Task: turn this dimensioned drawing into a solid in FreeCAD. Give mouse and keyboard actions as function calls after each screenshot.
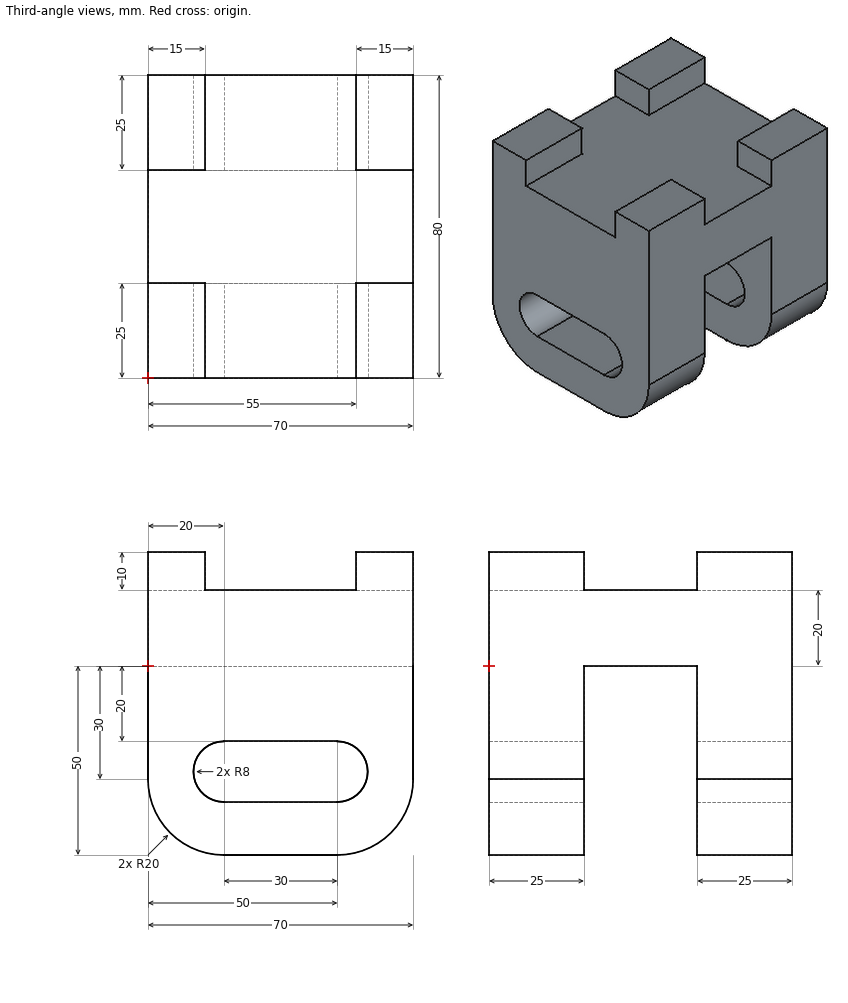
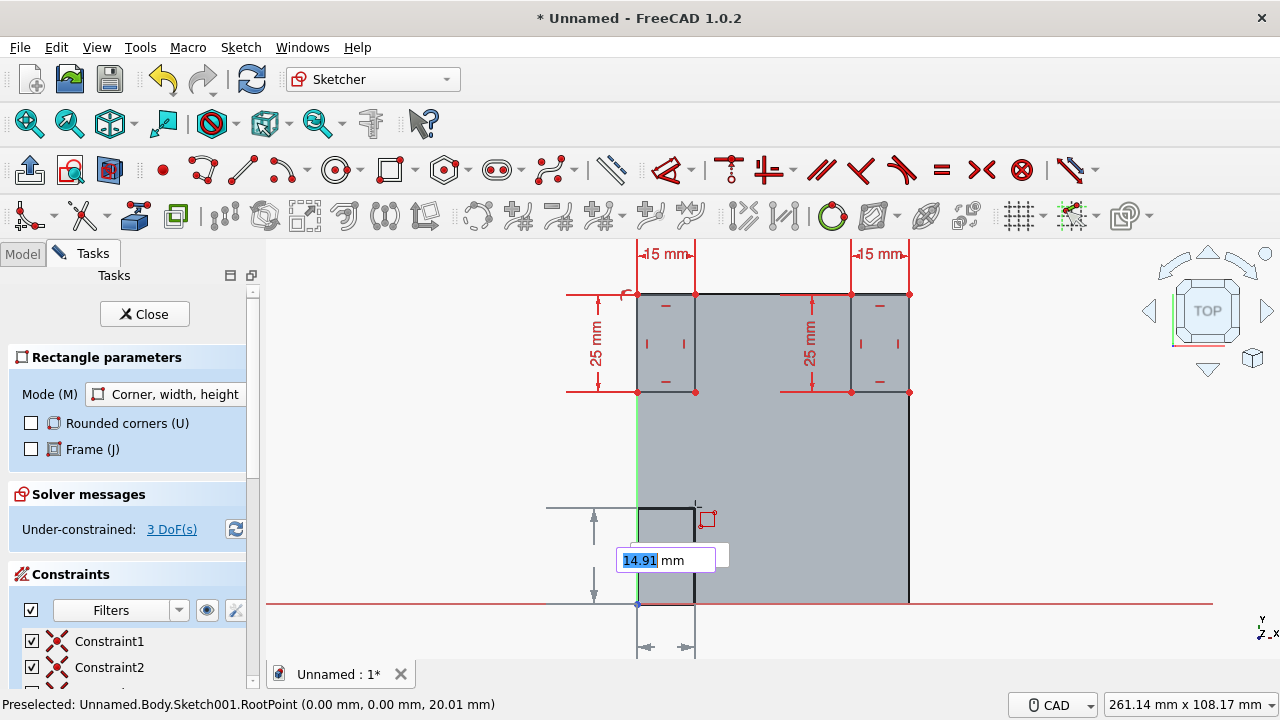
text(15)
key(Tab)
text(25)
key(Return)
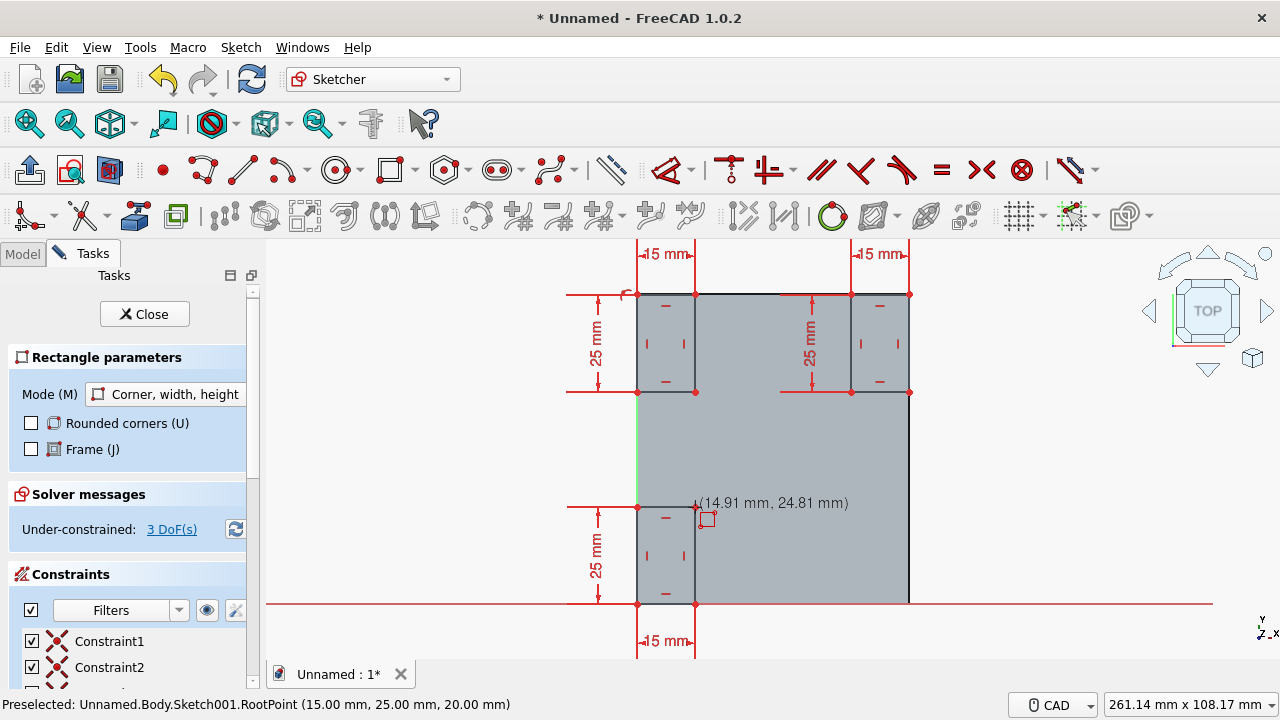
click(851, 507)
click(909, 604)
key(Escape)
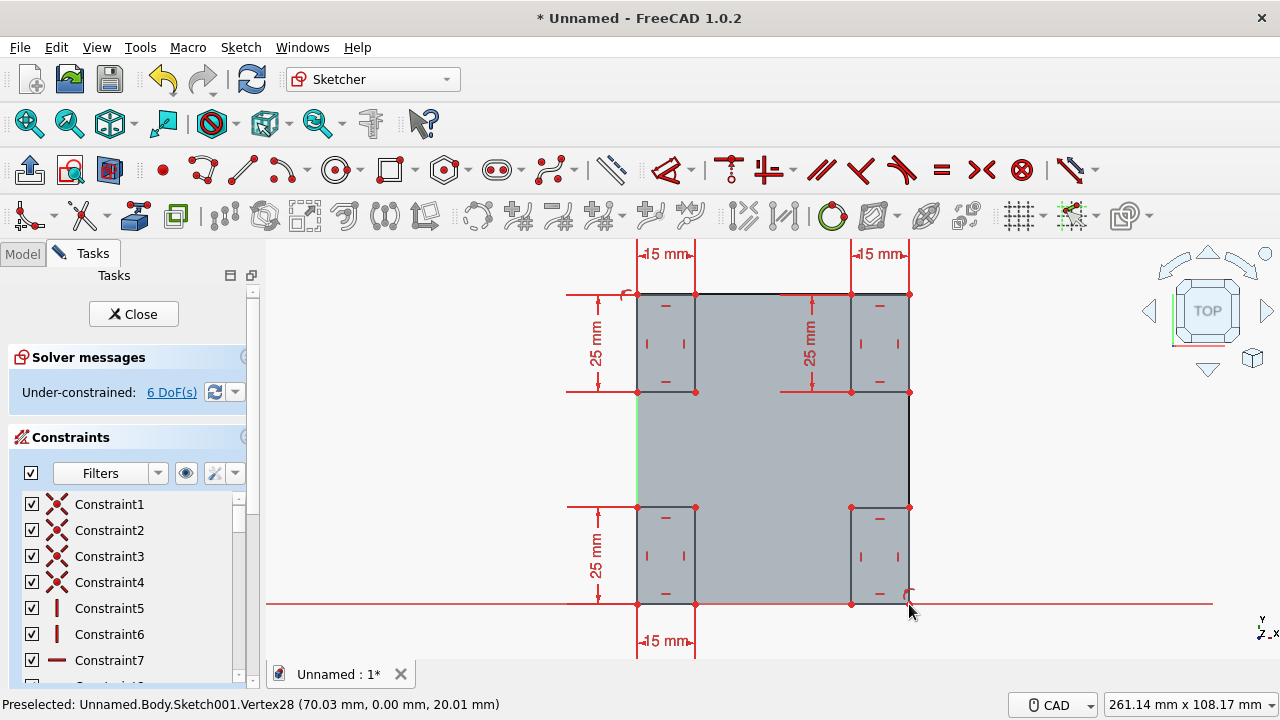
click(666, 170)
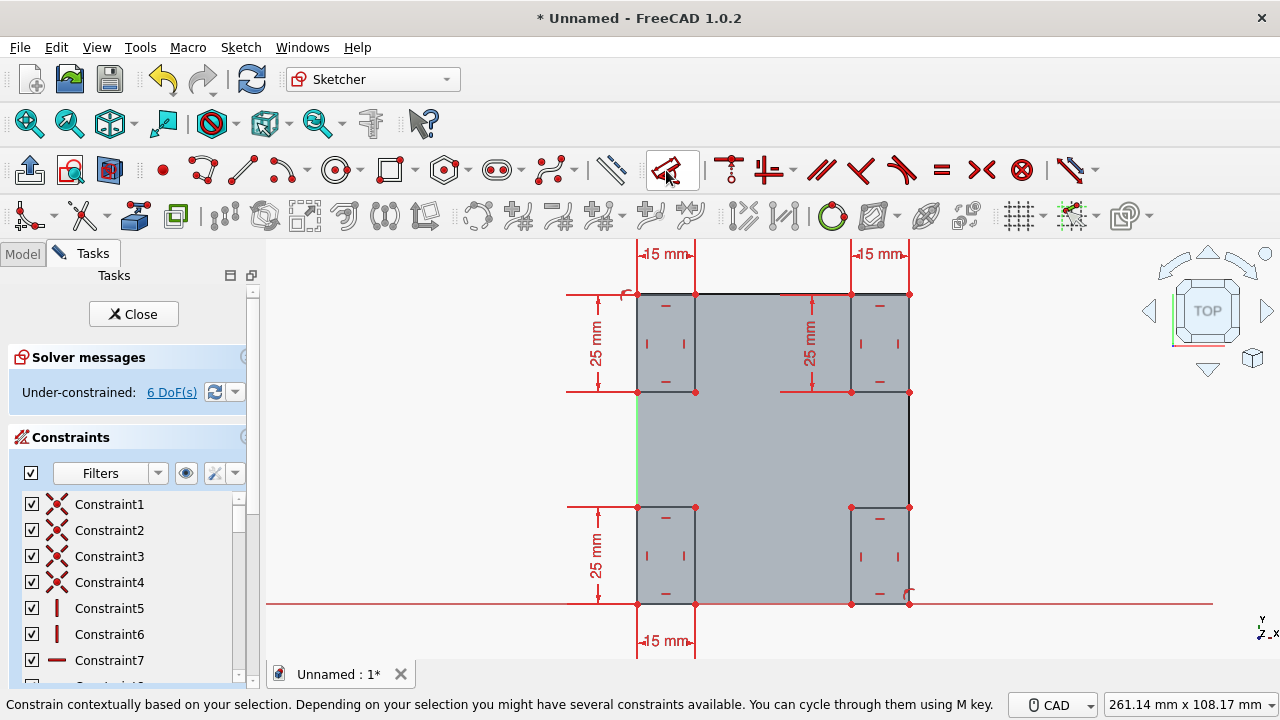
click(851, 537)
click(885, 556)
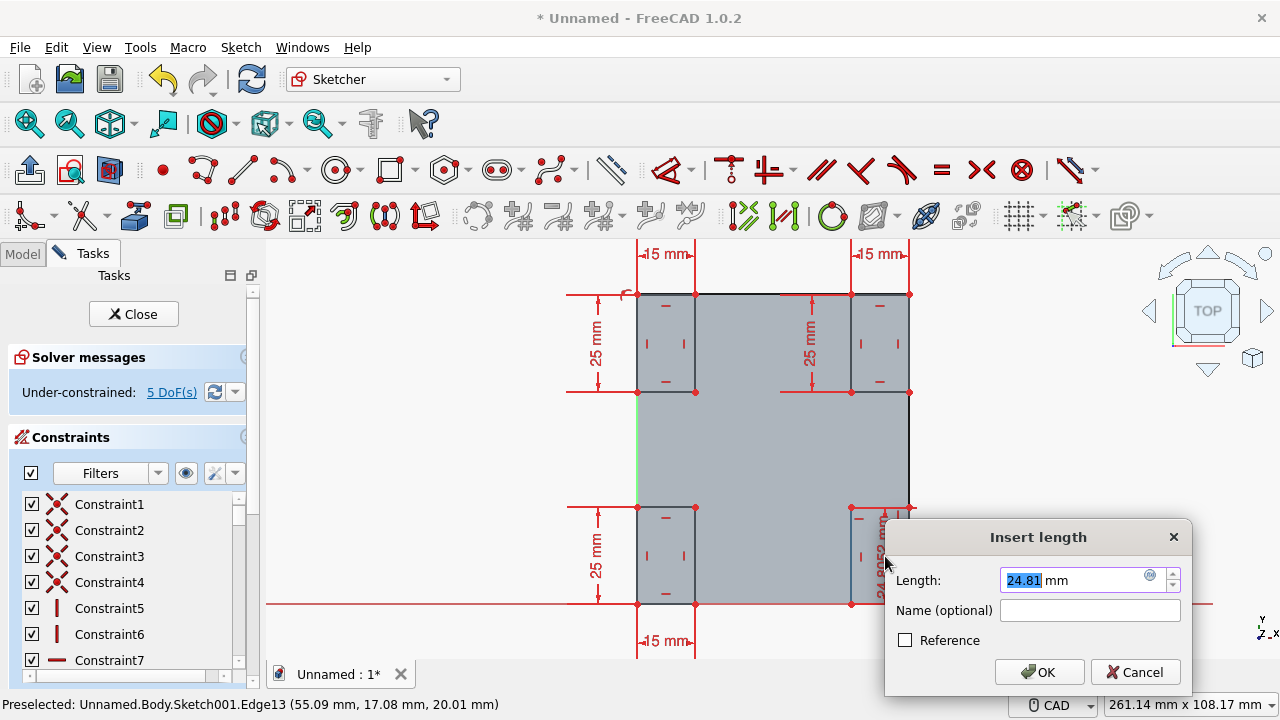
text(25)
key(Return)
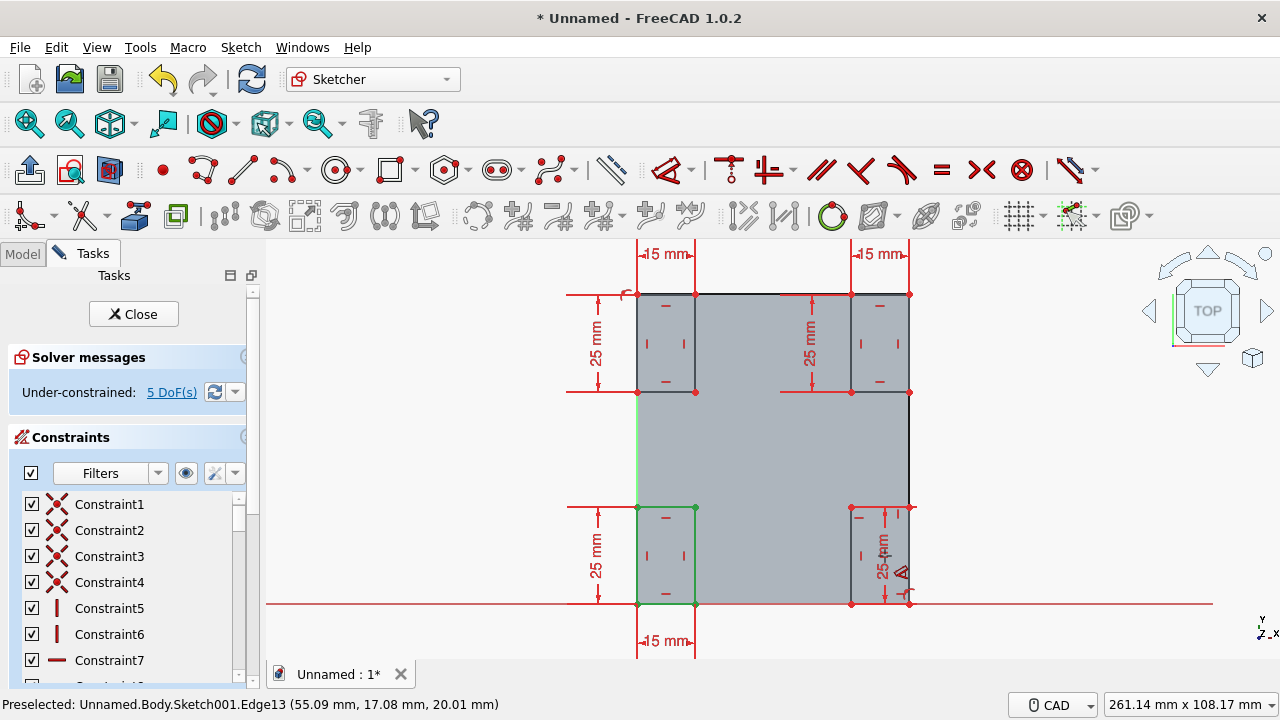
click(868, 604)
click(880, 522)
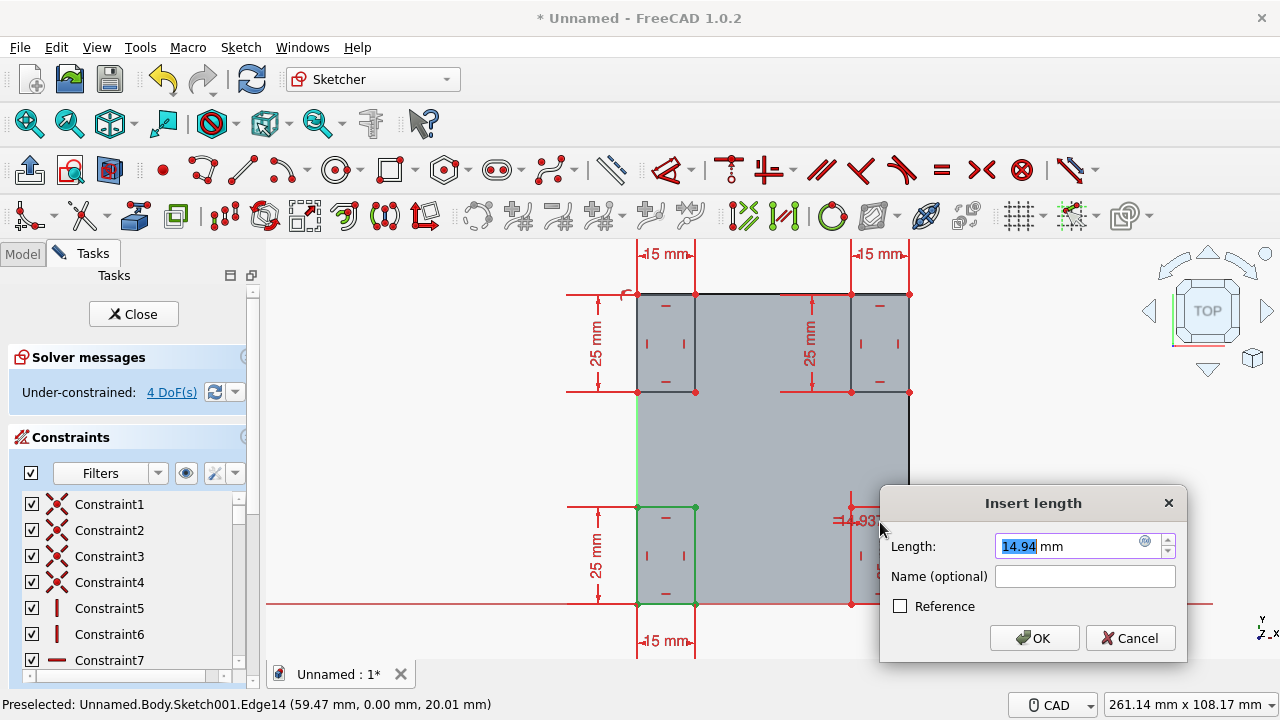
text(15)
key(Return)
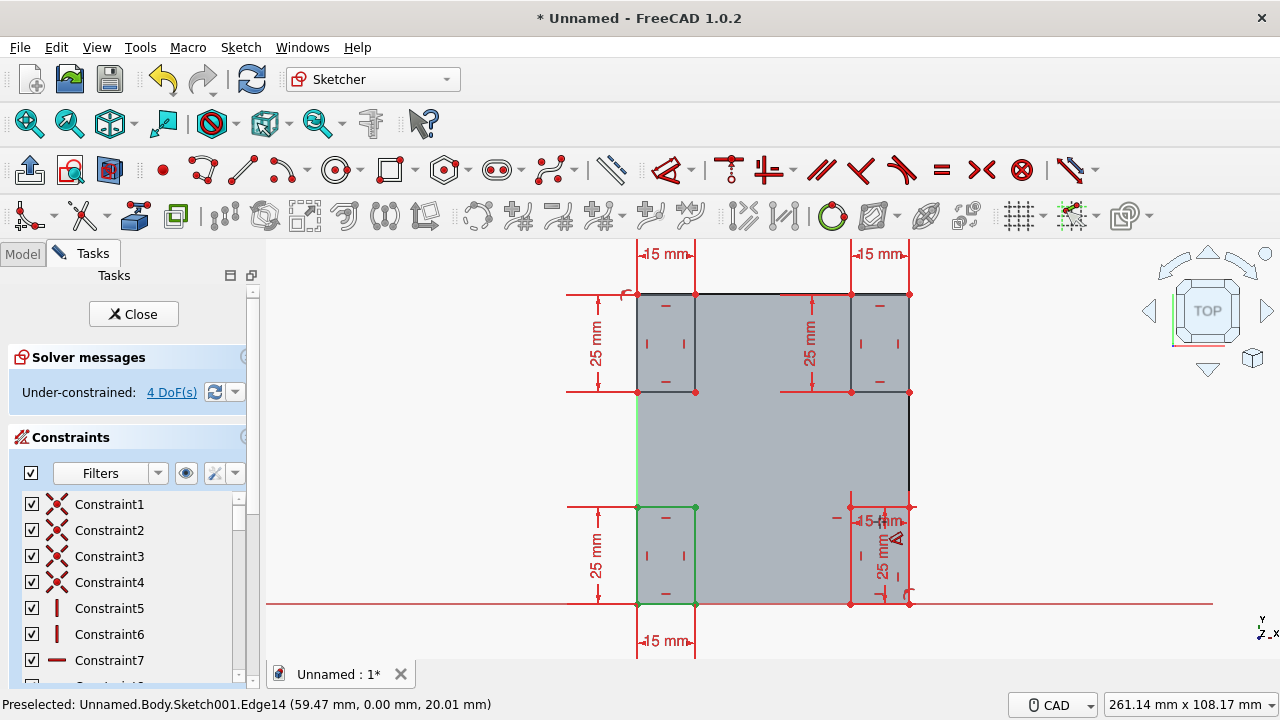
click(637, 295)
click(603, 450)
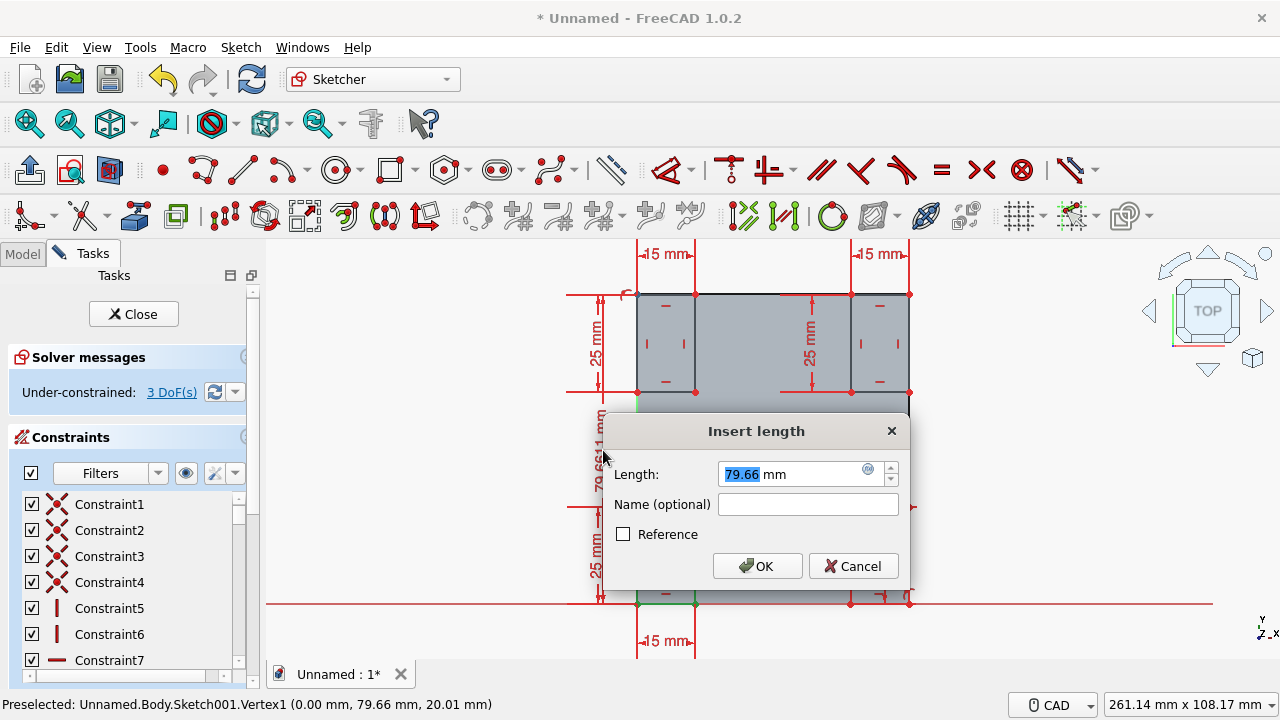
text(80)
key(Return)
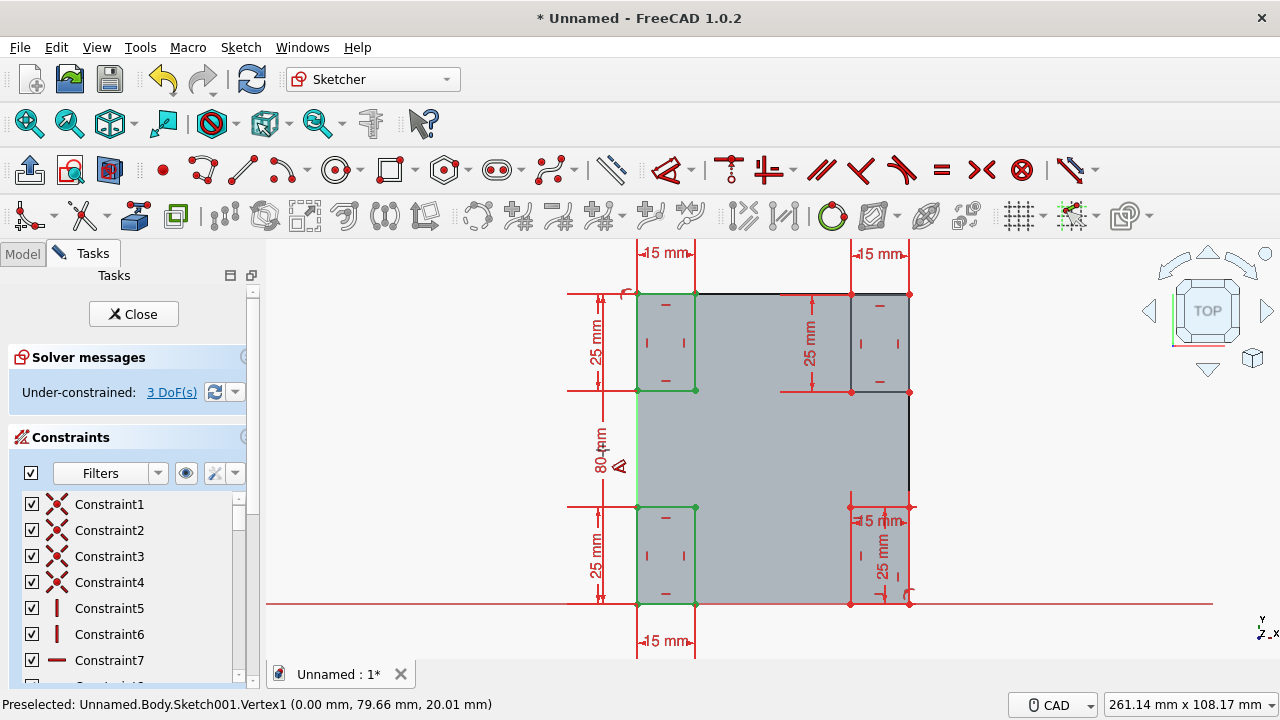
click(851, 295)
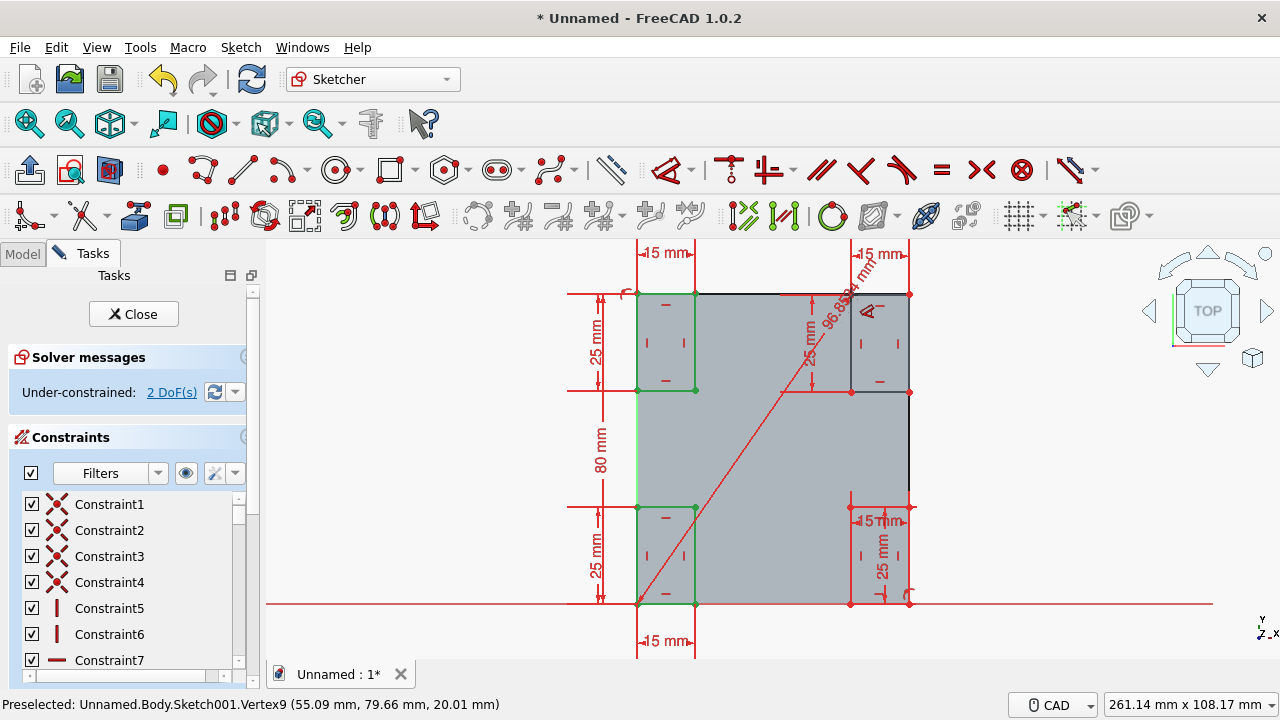
key(Escape)
key(Escape)